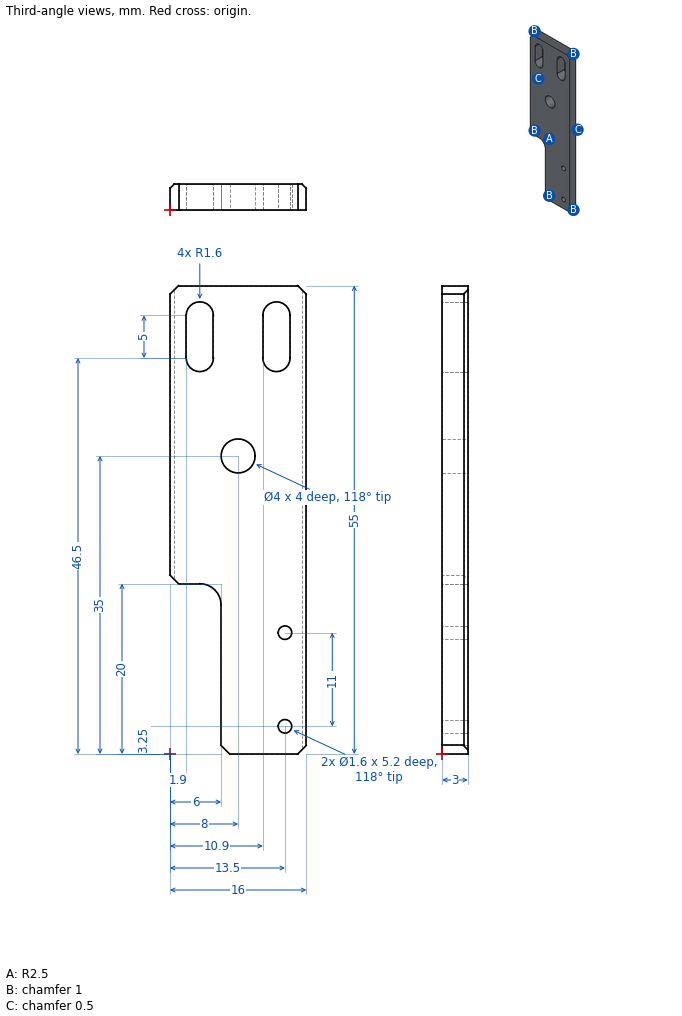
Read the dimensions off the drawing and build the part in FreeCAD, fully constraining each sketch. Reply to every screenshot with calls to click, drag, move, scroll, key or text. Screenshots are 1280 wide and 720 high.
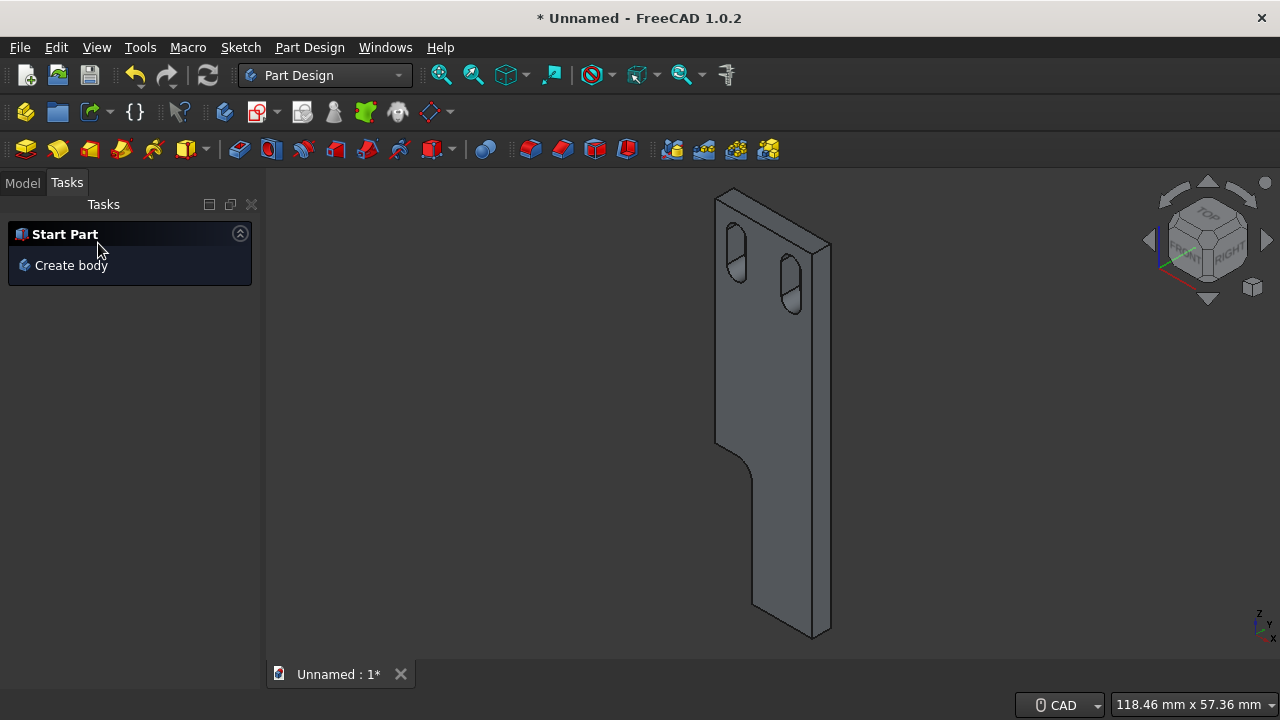
click(821, 248)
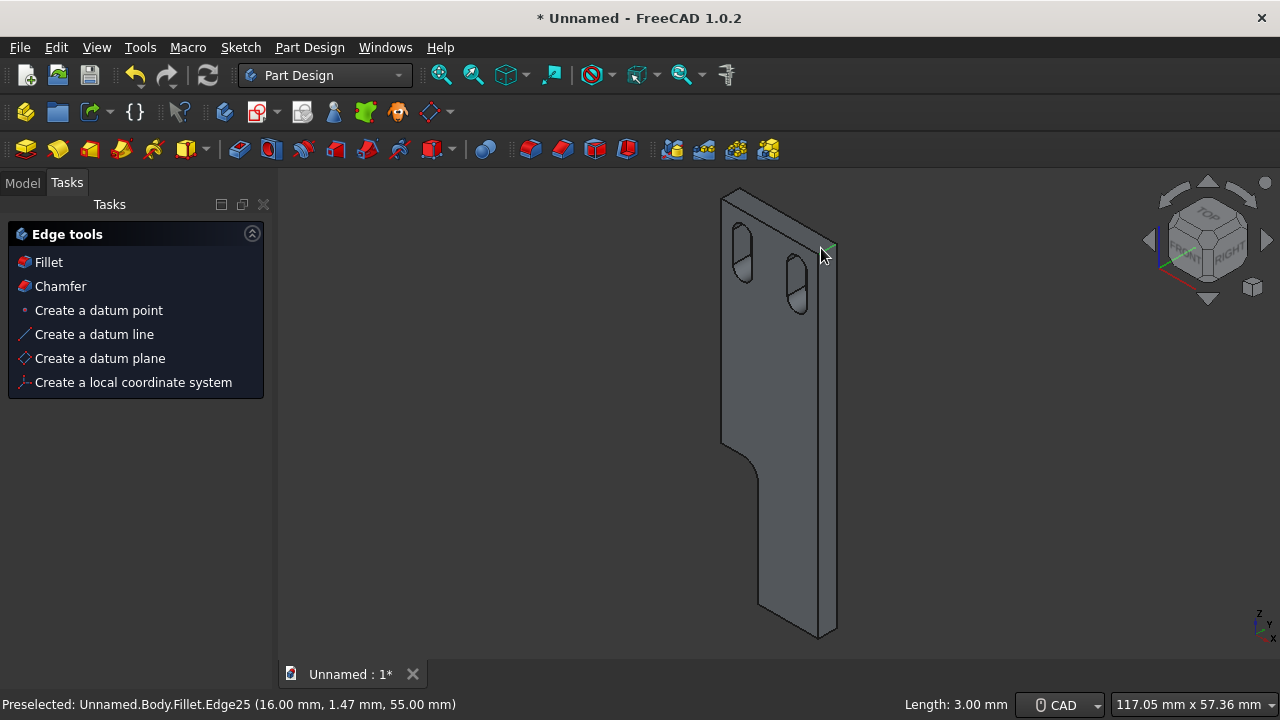
key(2)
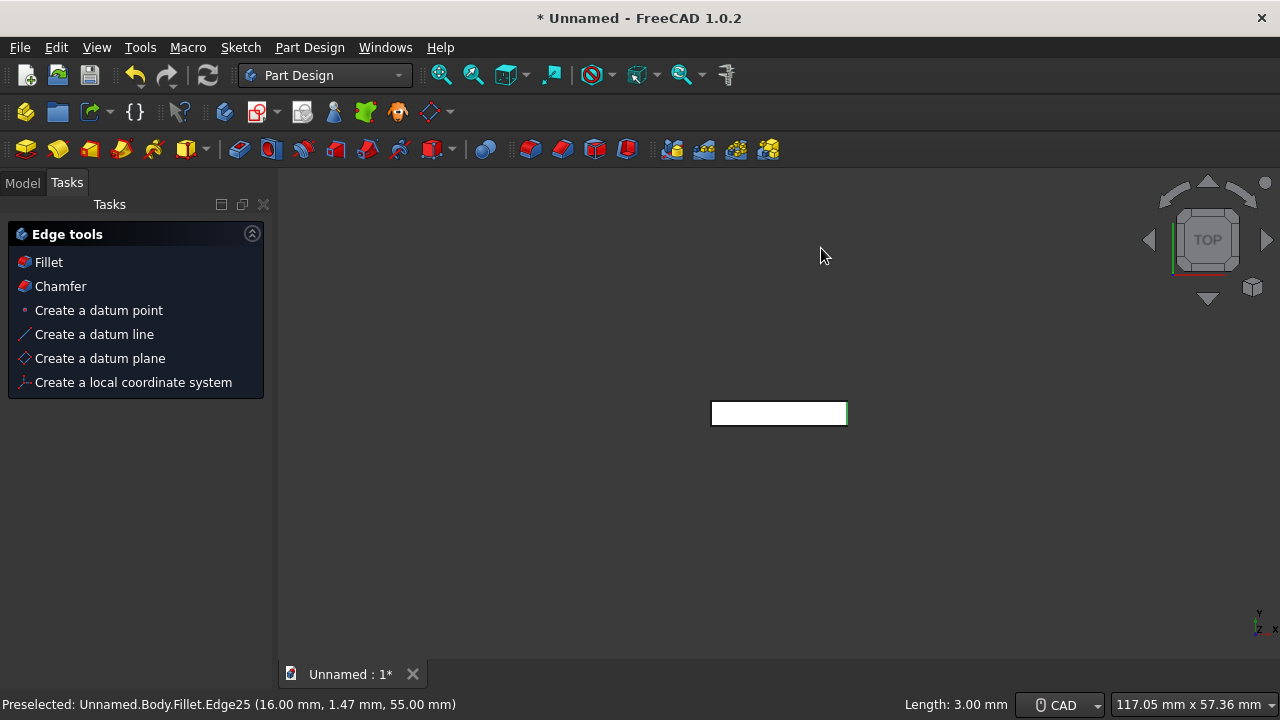
click(442, 76)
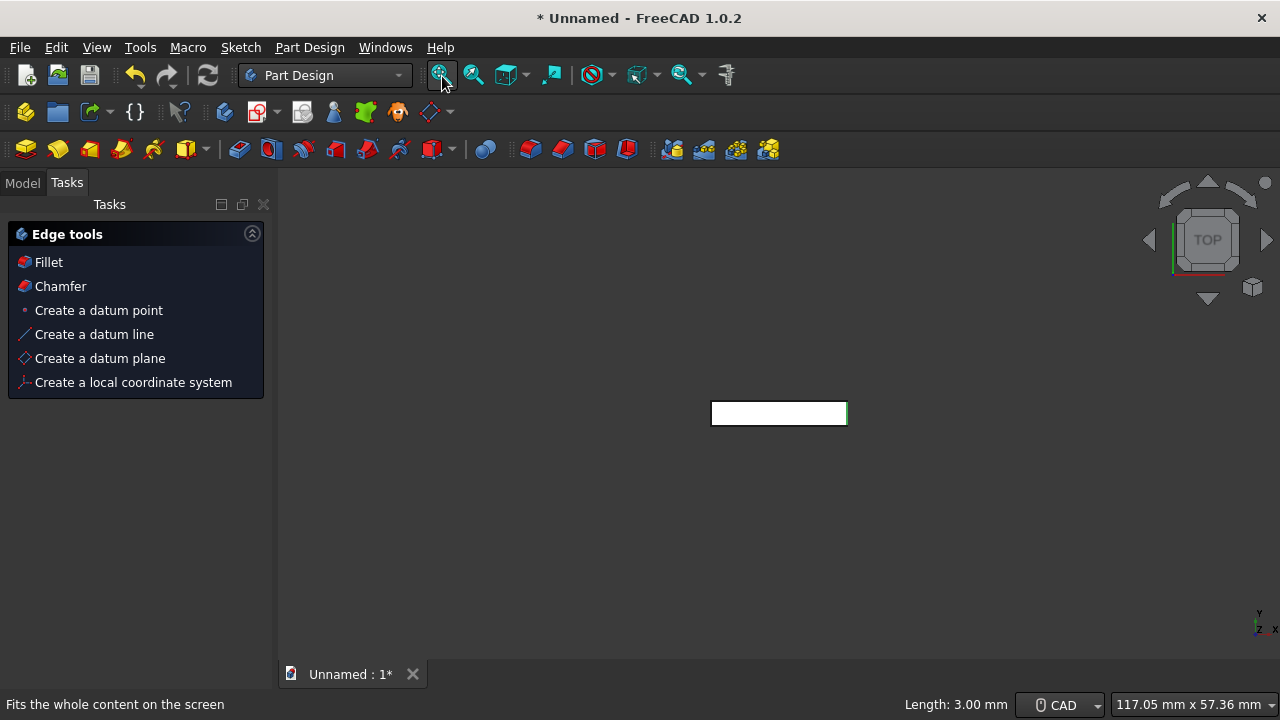
click(711, 412, ctrl)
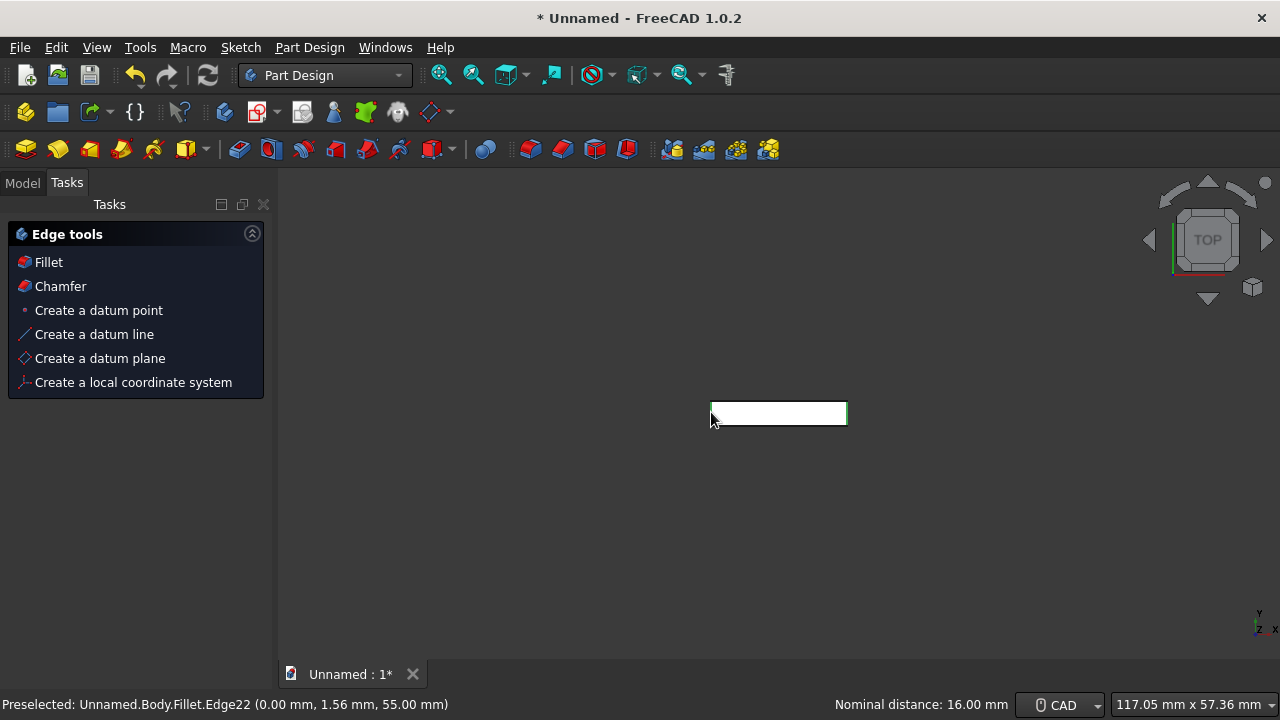
key(0)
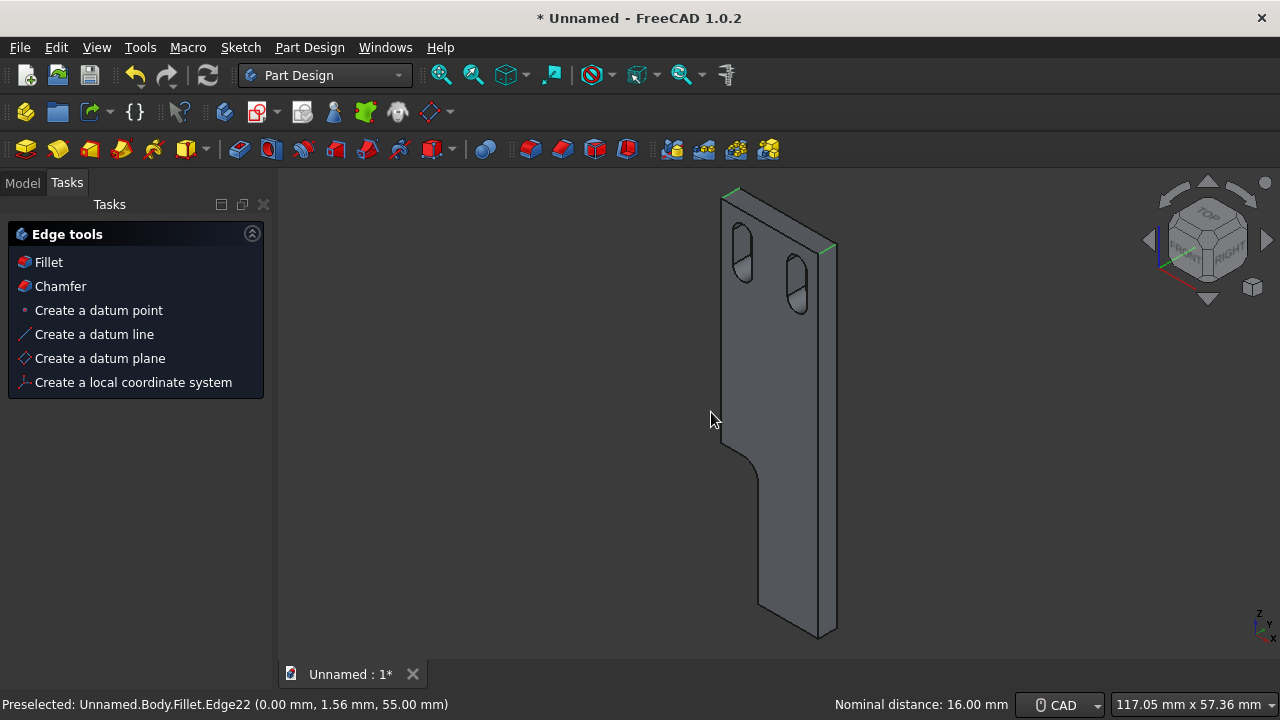
key(1)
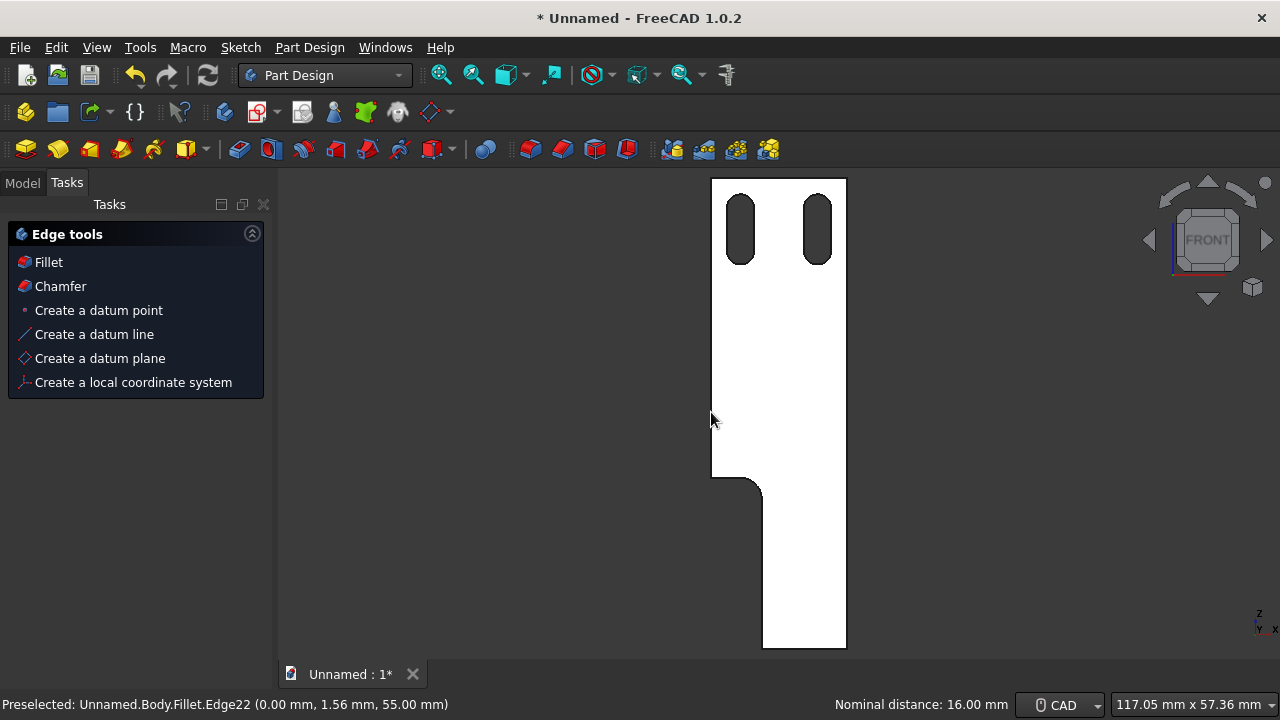
key(3)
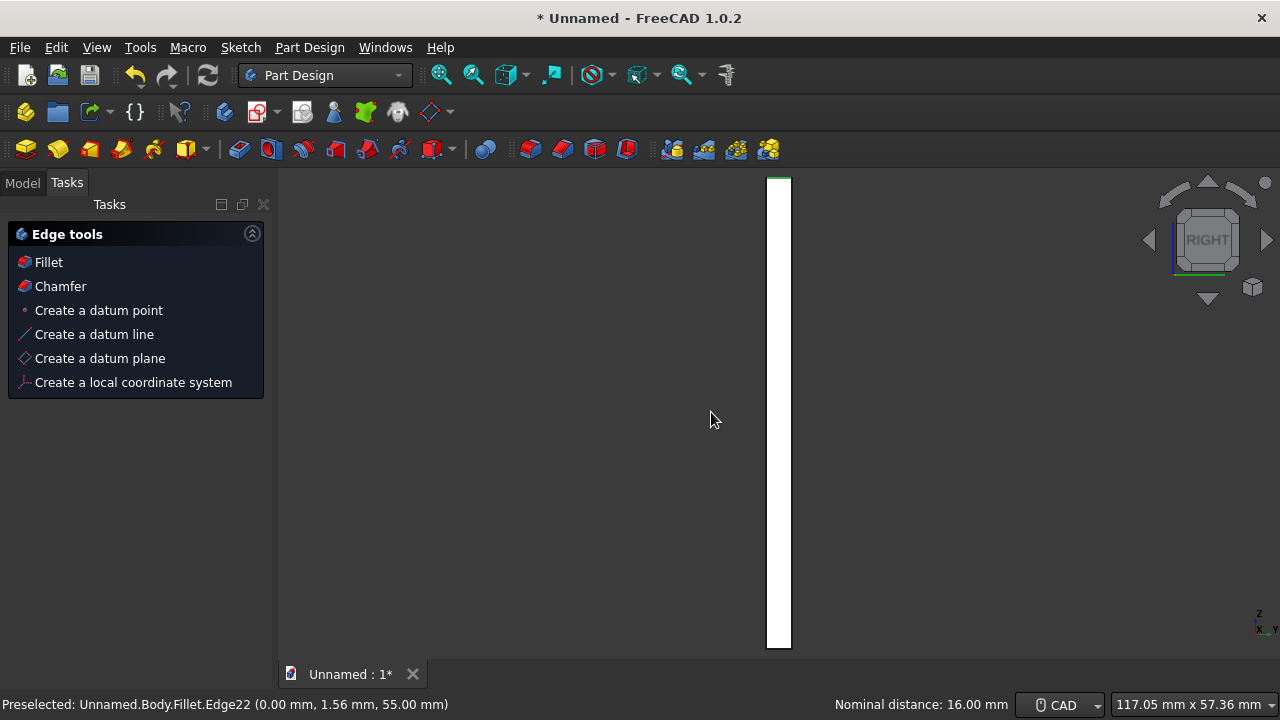
key(5)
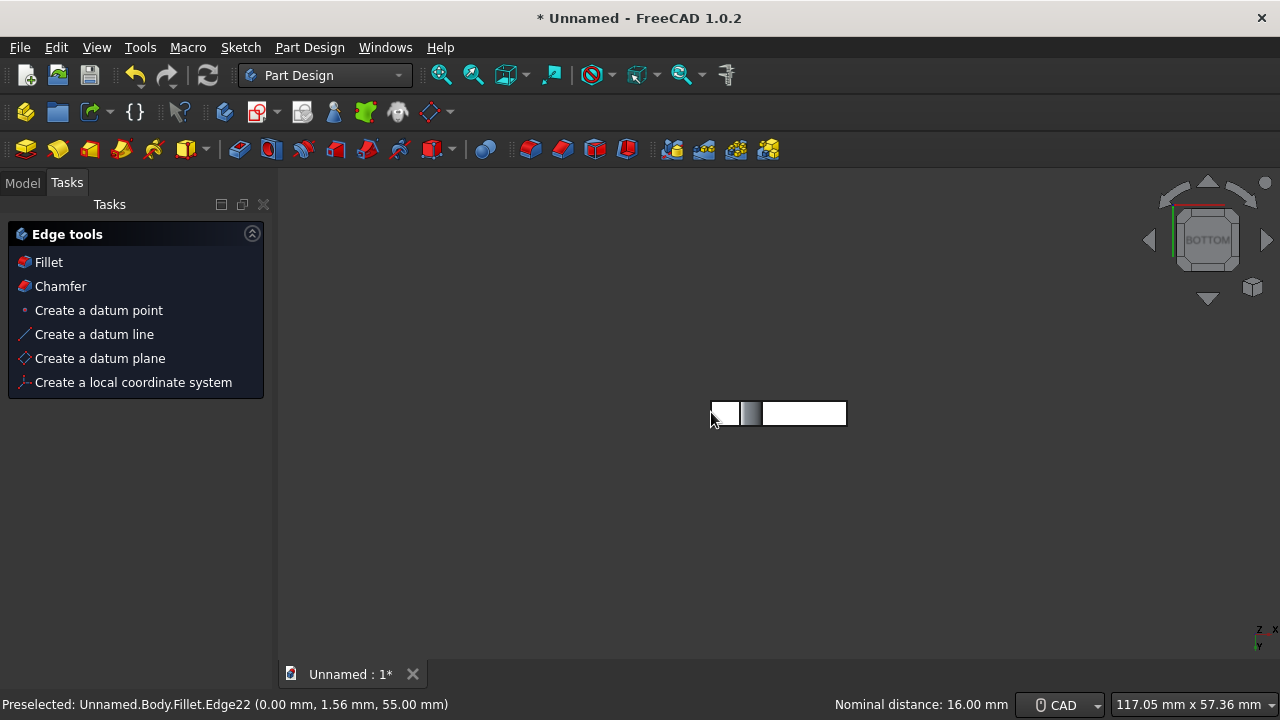
click(442, 76)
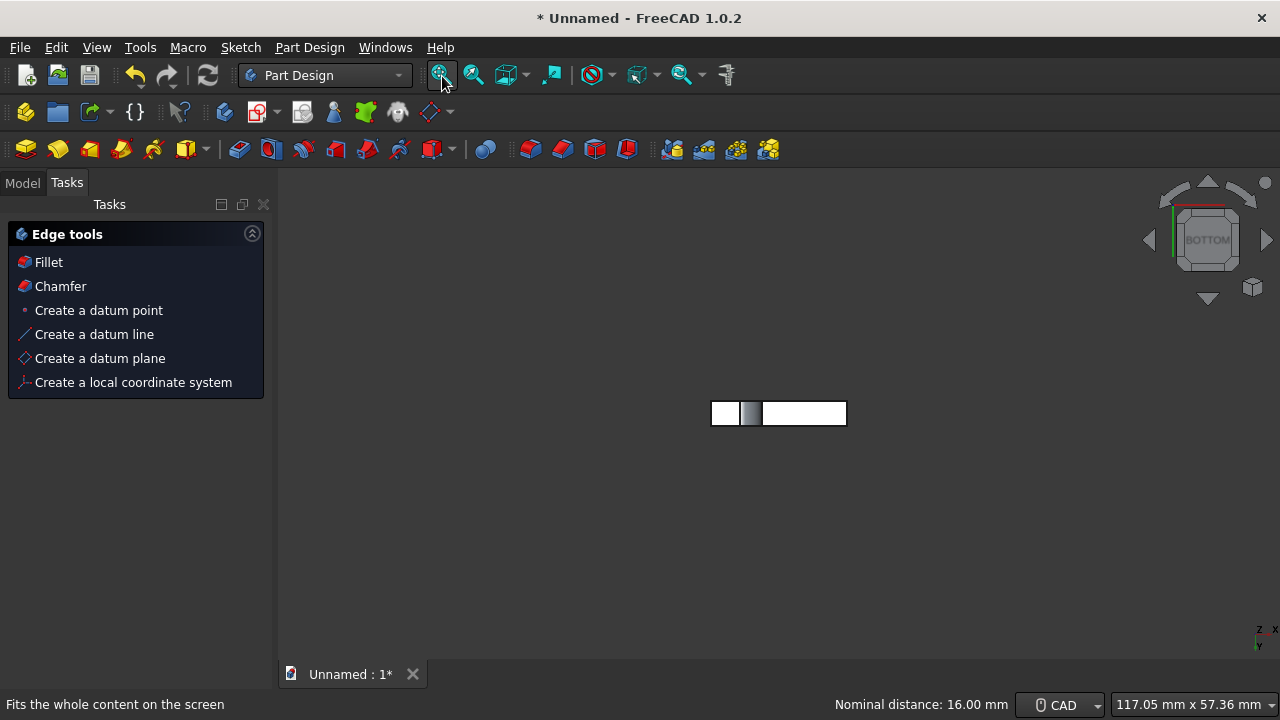
click(711, 413, ctrl)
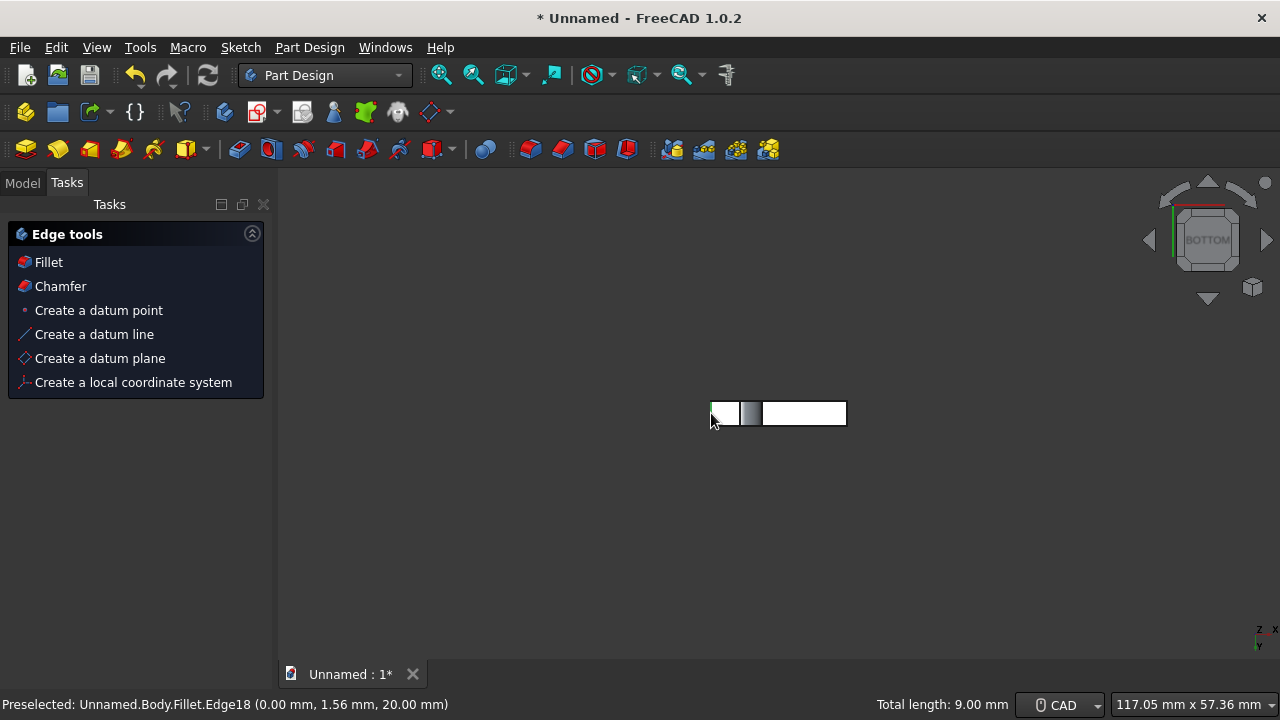
click(762, 413, ctrl)